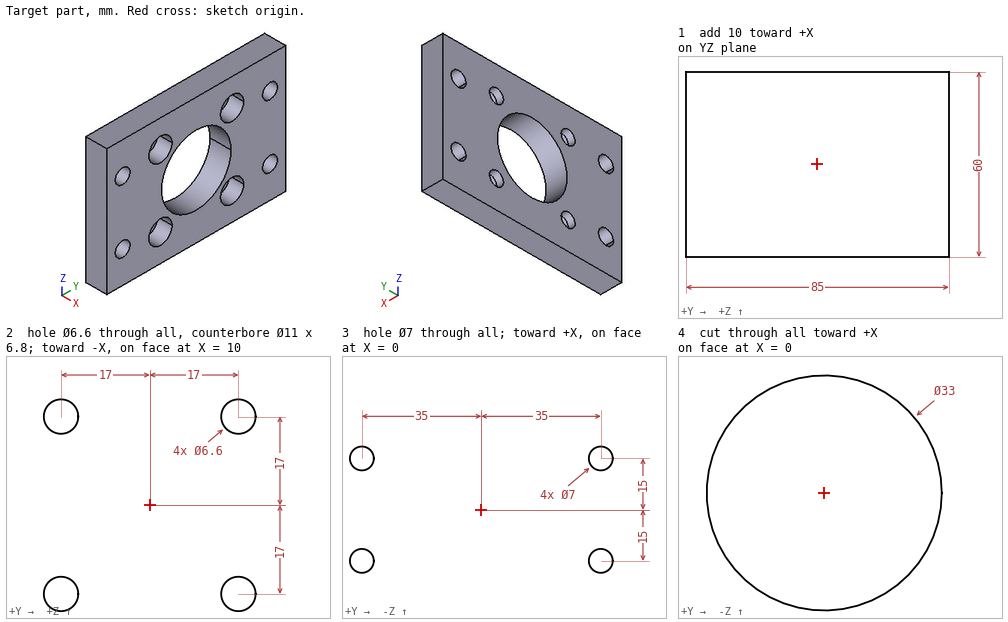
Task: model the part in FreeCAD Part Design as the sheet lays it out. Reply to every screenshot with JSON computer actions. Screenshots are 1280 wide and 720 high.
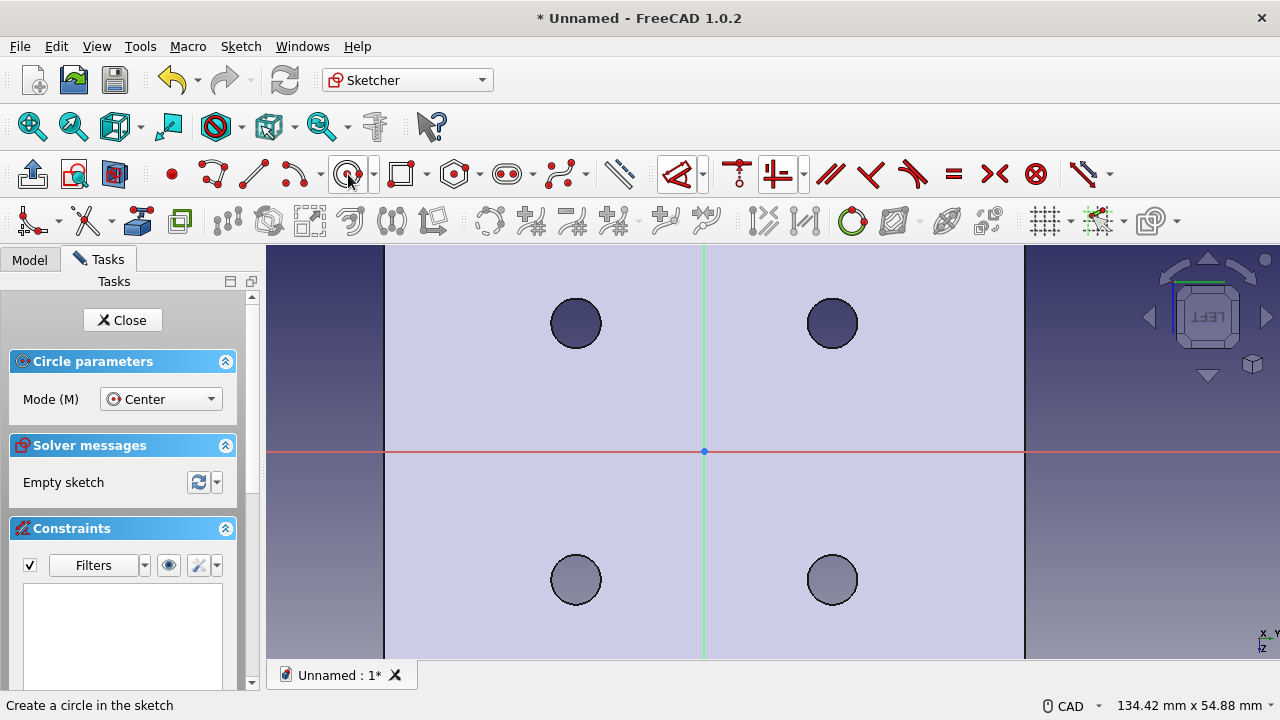
{"action": "left_click", "coordinate": [968, 338]}
{"action": "left_click", "coordinate": [987, 320]}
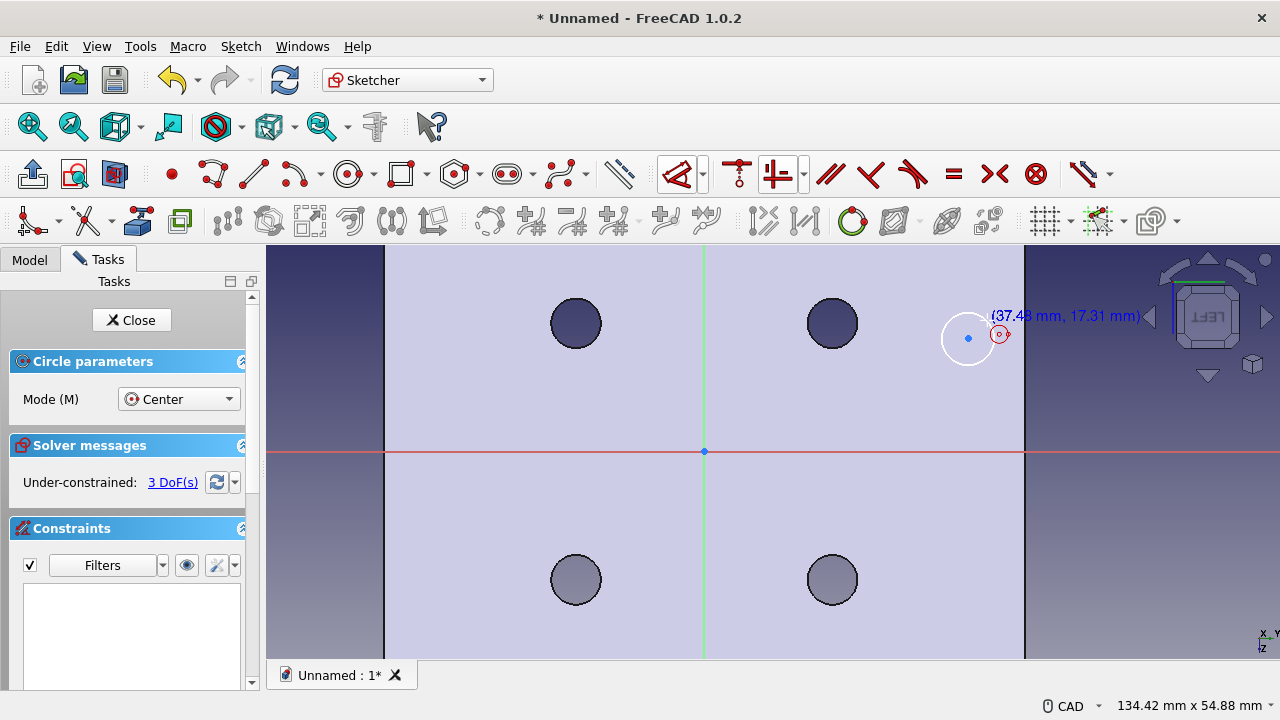
{"action": "left_click", "coordinate": [968, 565]}
{"action": "left_click", "coordinate": [987, 546]}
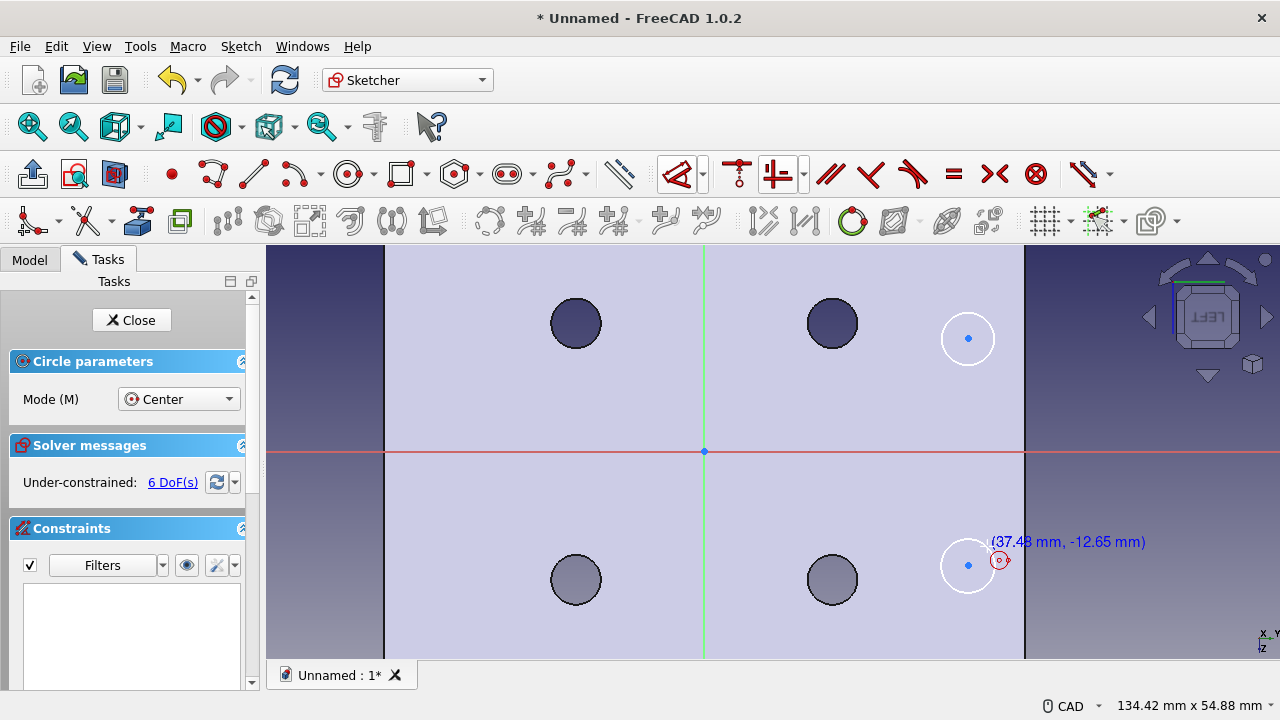
{"action": "left_click", "coordinate": [440, 338]}
{"action": "left_click", "coordinate": [459, 320]}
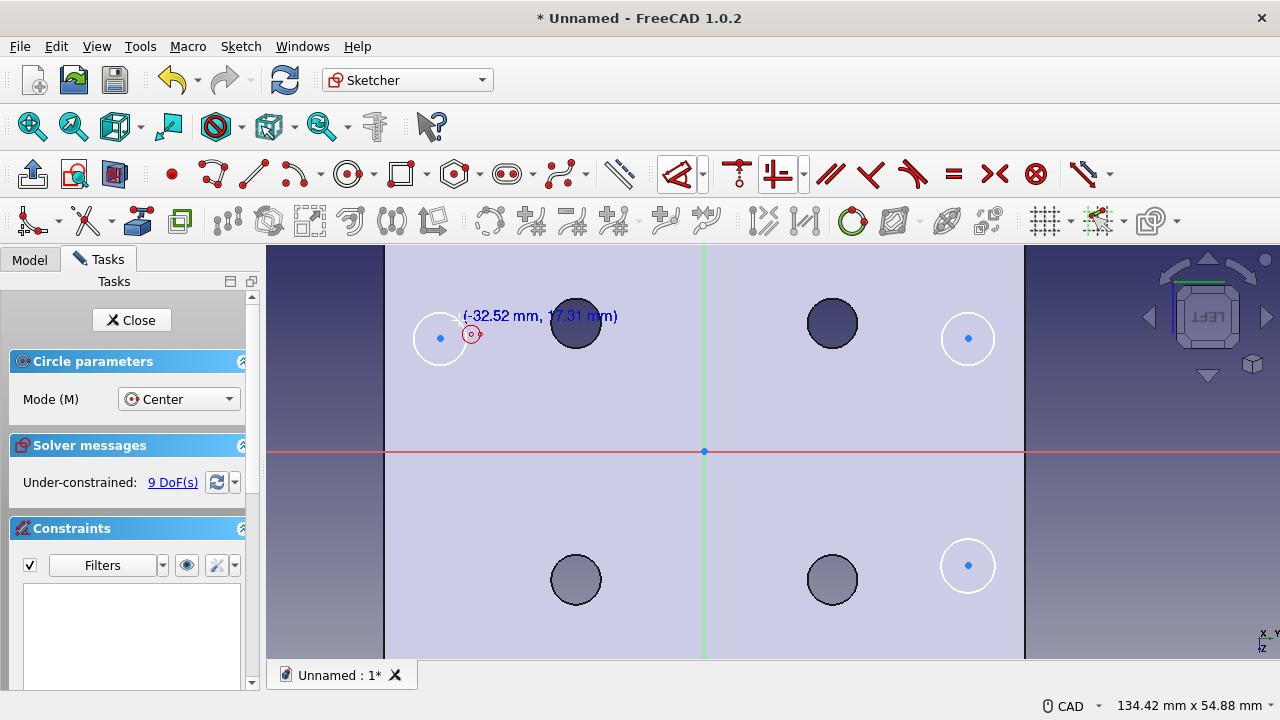
{"action": "left_click", "coordinate": [440, 565]}
{"action": "left_click", "coordinate": [459, 546]}
{"action": "key", "text": "Escape"}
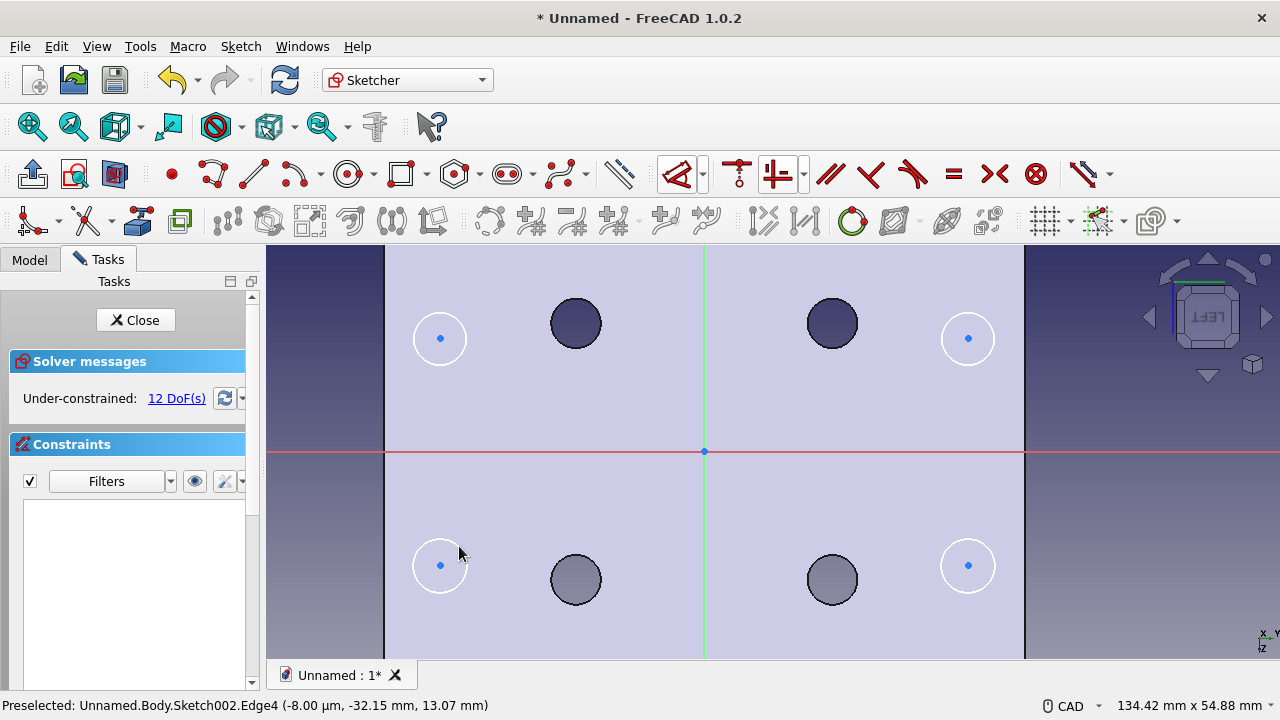
{"action": "left_click", "coordinate": [986, 320]}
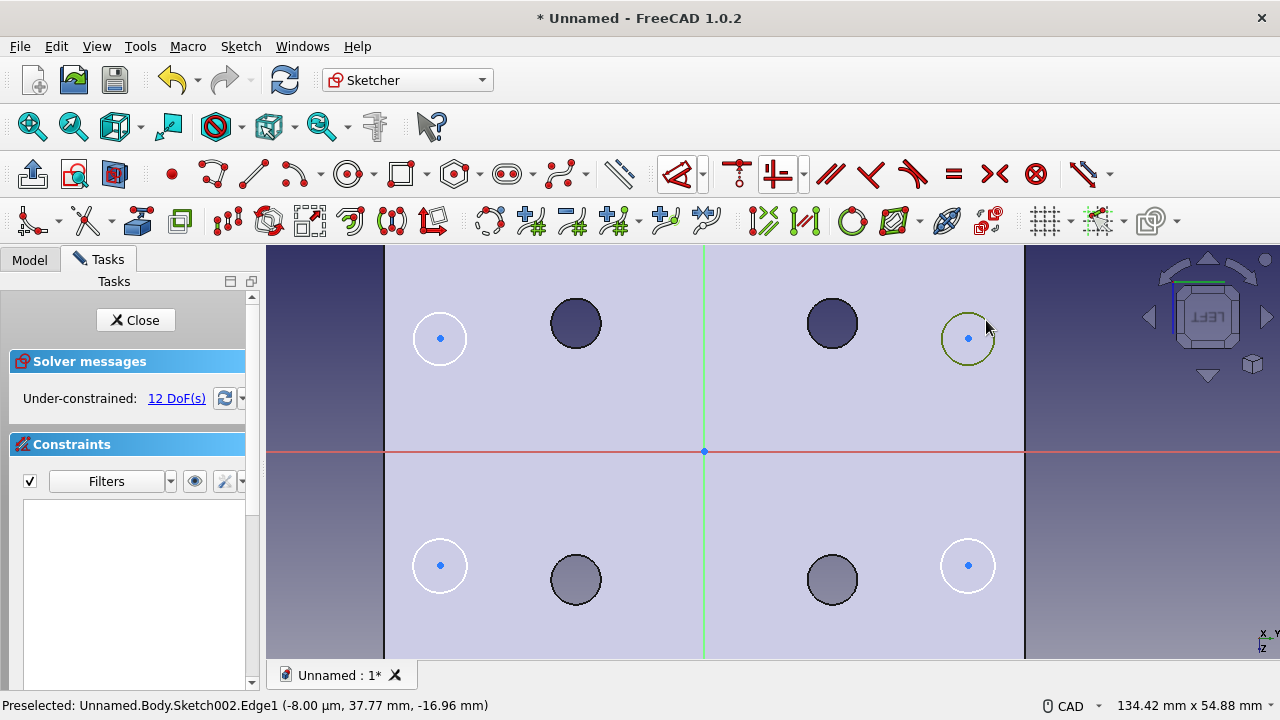
{"action": "left_click", "coordinate": [987, 547]}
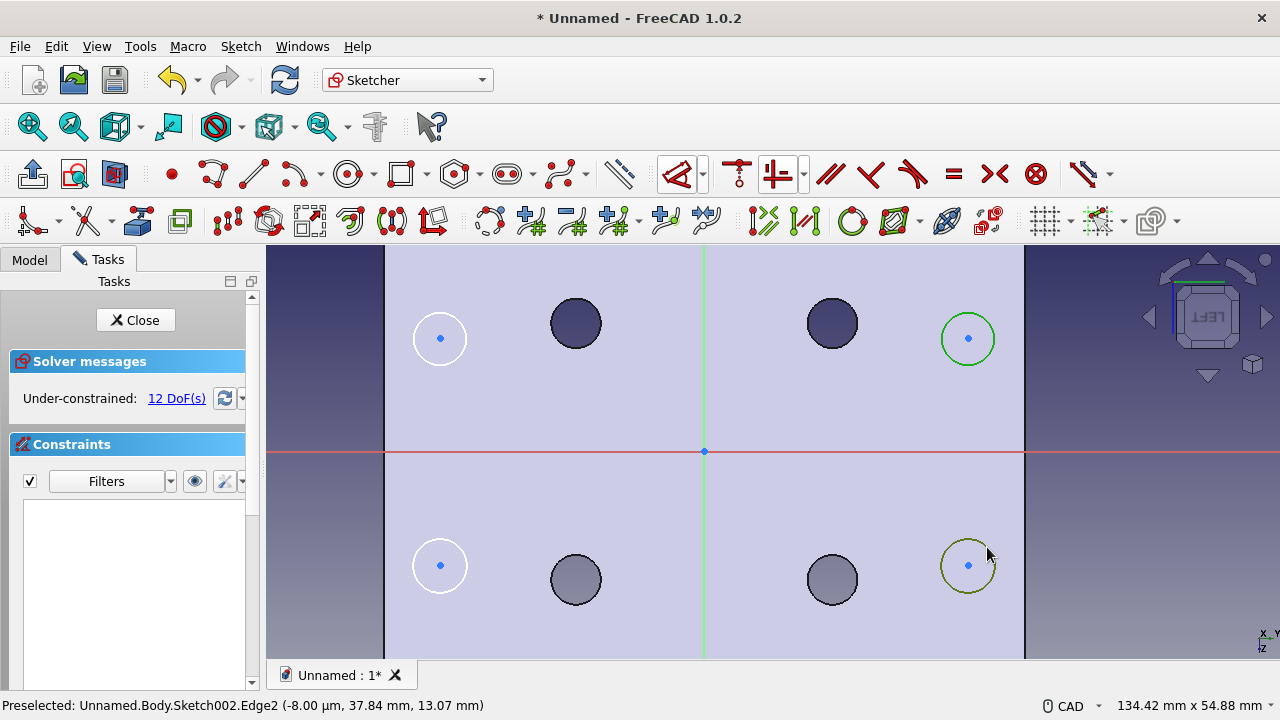
{"action": "left_click", "coordinate": [458, 320]}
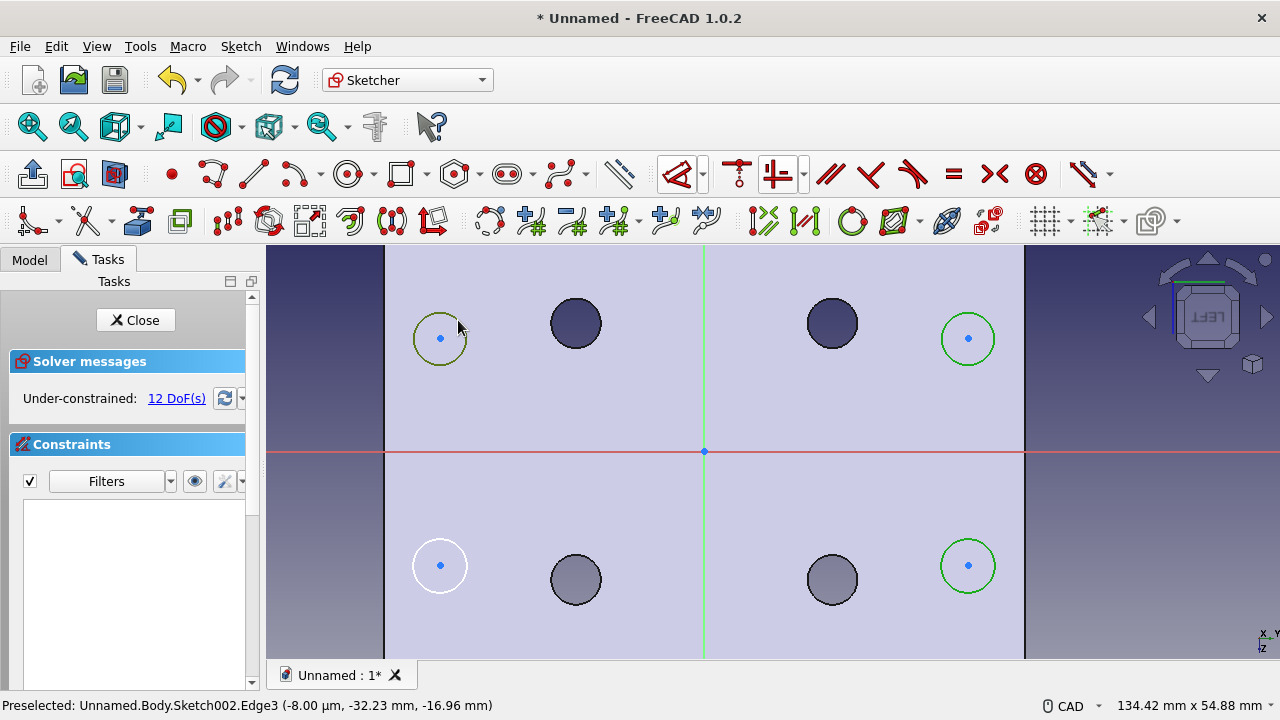
{"action": "left_click", "coordinate": [459, 547]}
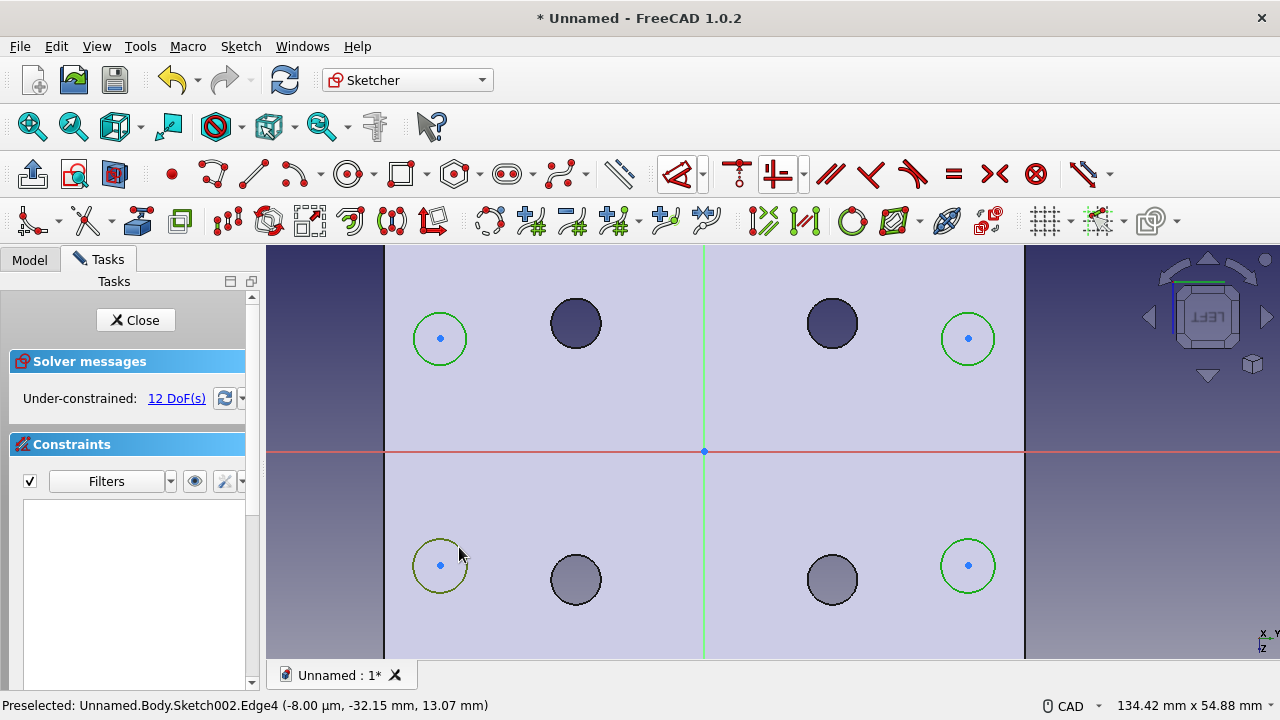
{"action": "key", "text": "e"}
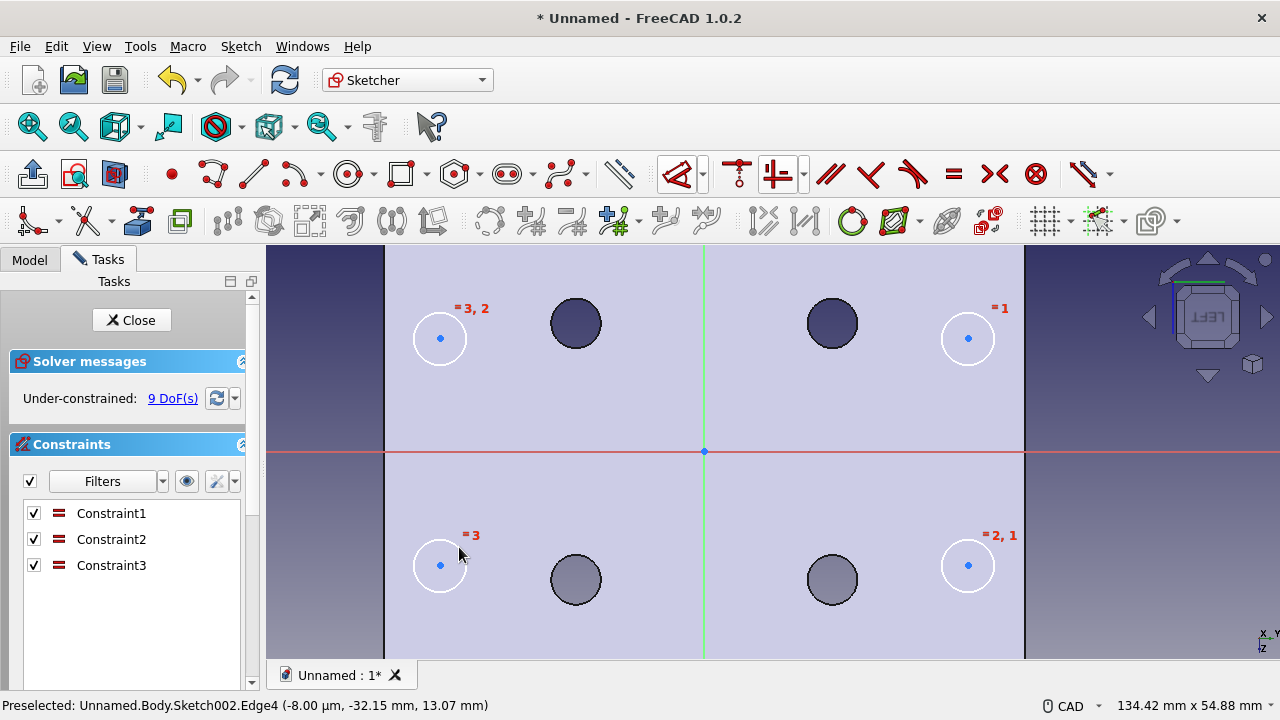
{"action": "left_click", "coordinate": [968, 339]}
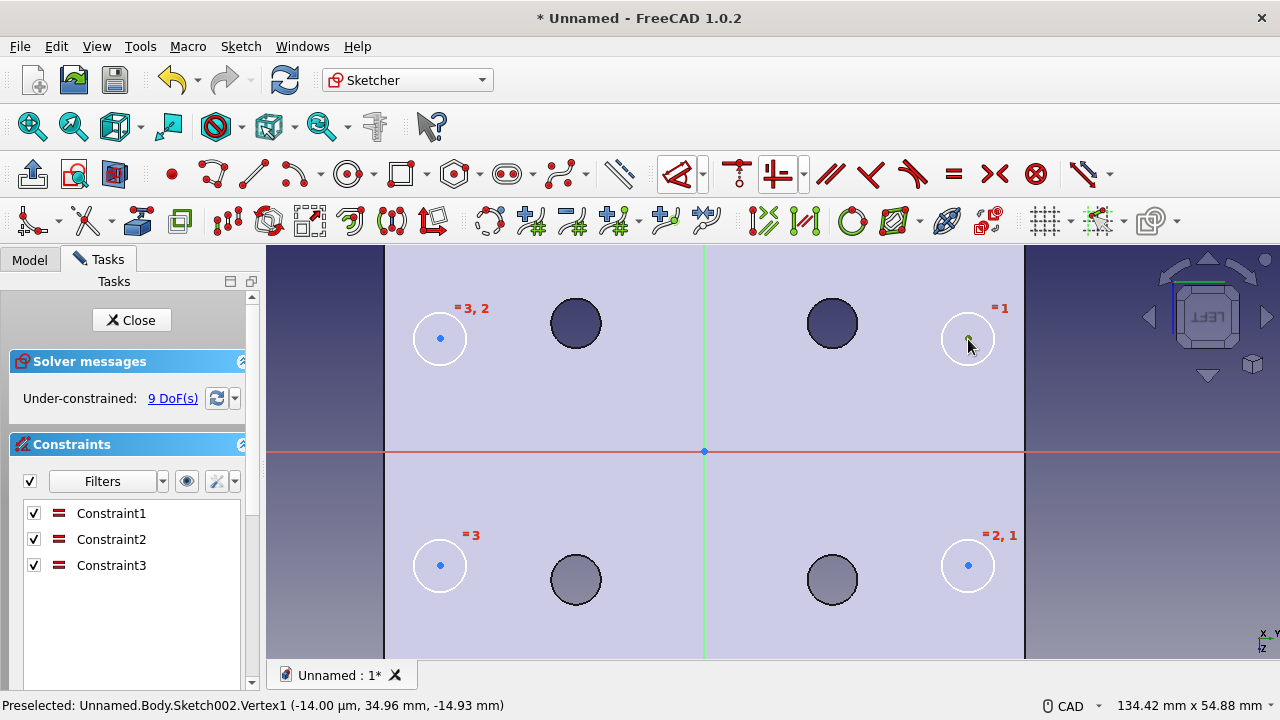
{"action": "left_click", "coordinate": [968, 566]}